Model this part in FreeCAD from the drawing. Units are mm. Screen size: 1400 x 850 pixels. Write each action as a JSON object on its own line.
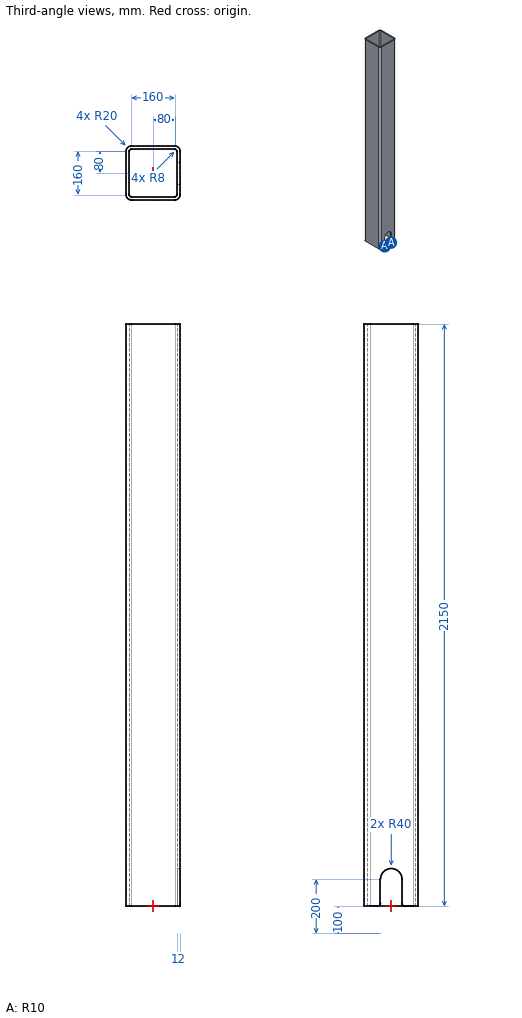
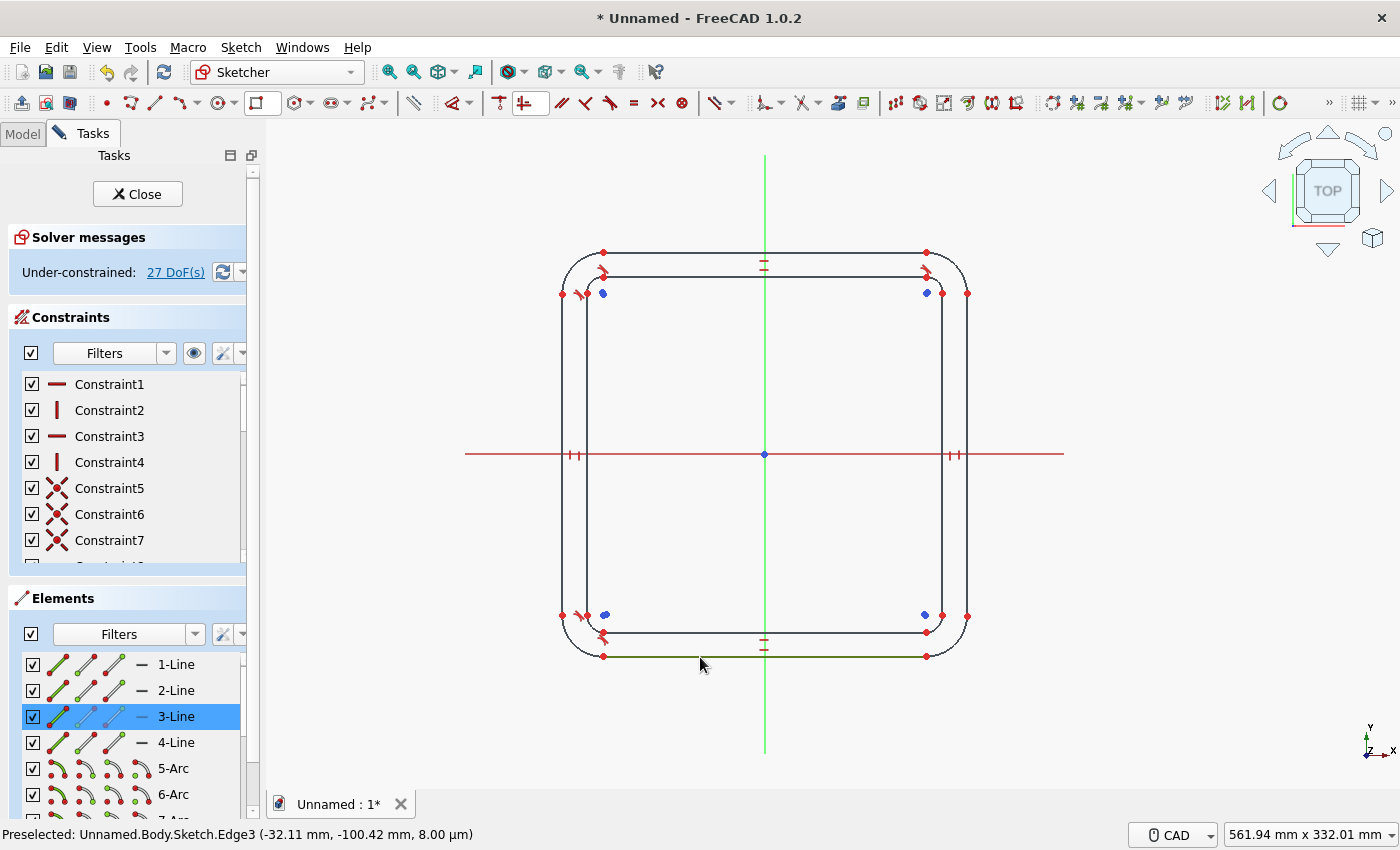
{"action": "left_click", "coordinate": [944, 652]}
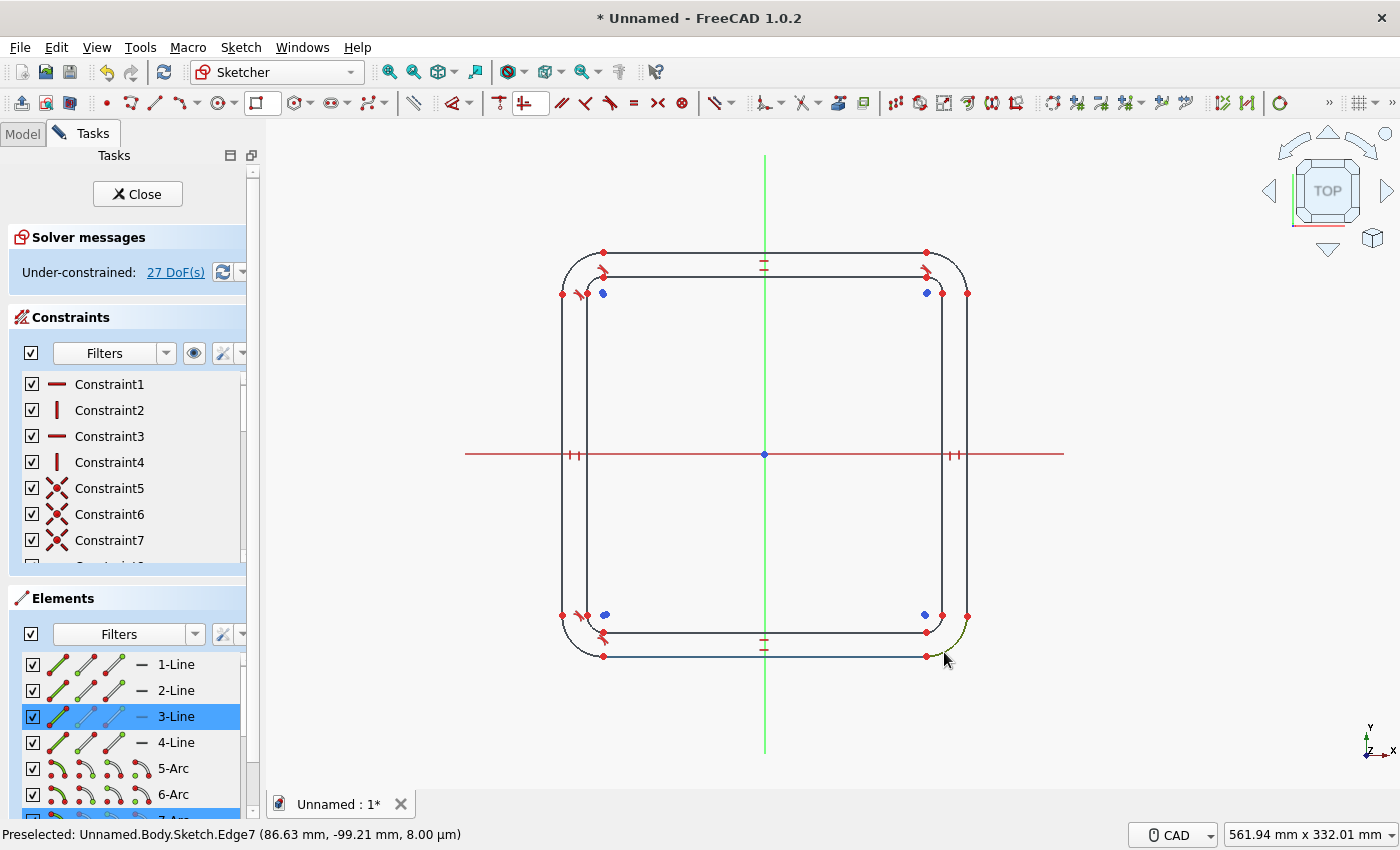
{"action": "left_click", "coordinate": [610, 104]}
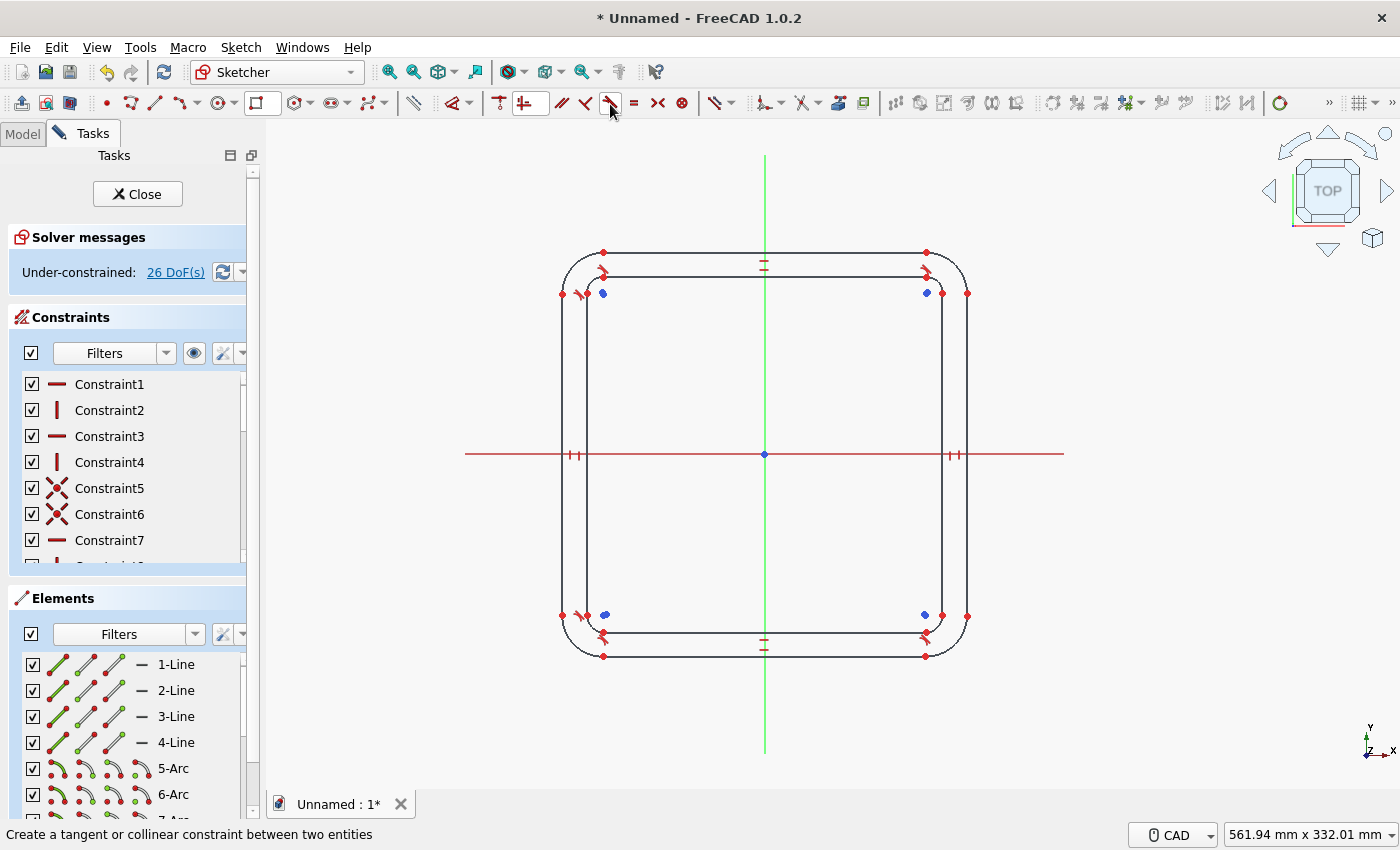
{"action": "left_click", "coordinate": [967, 520]}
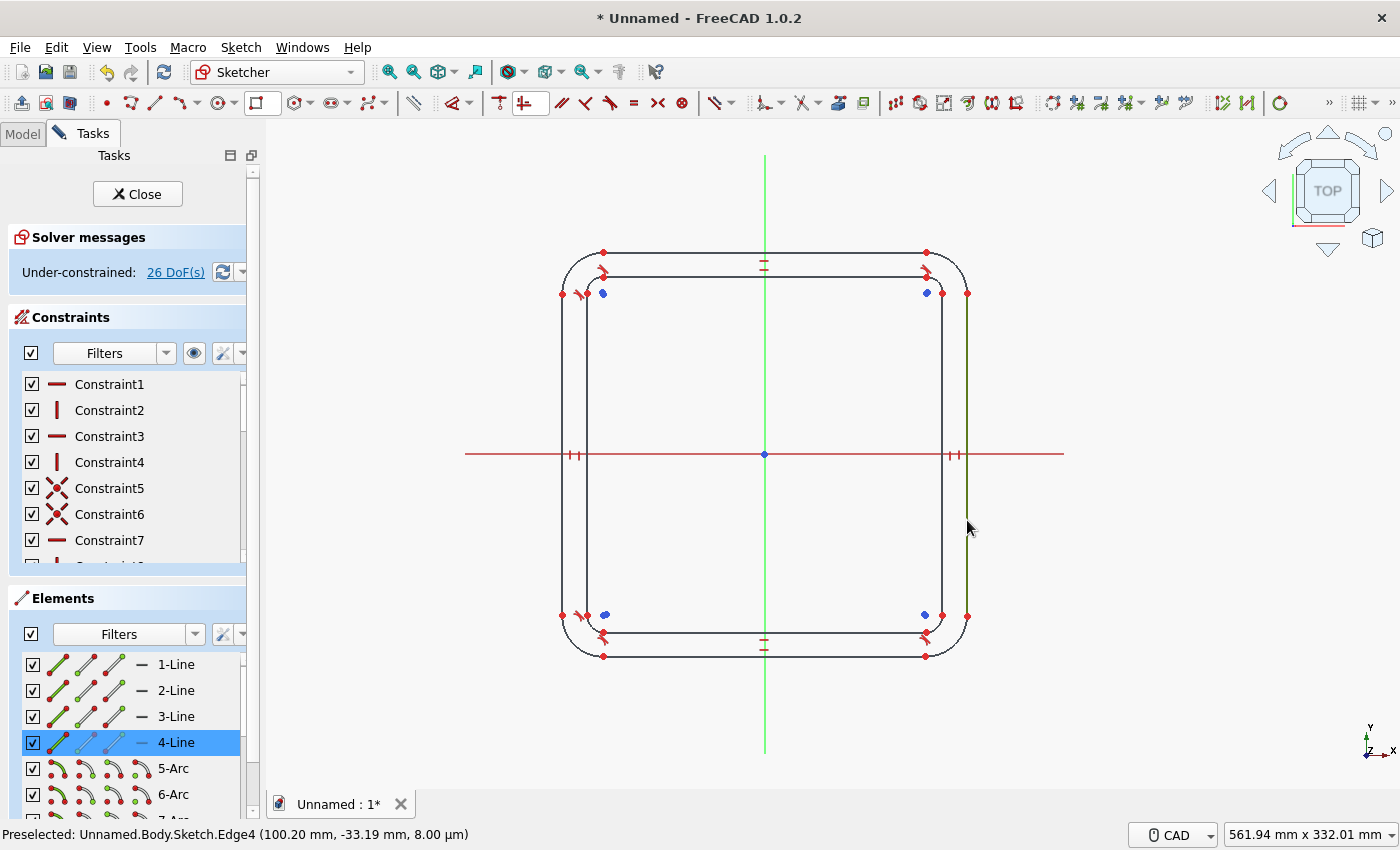
{"action": "left_click", "coordinate": [944, 652]}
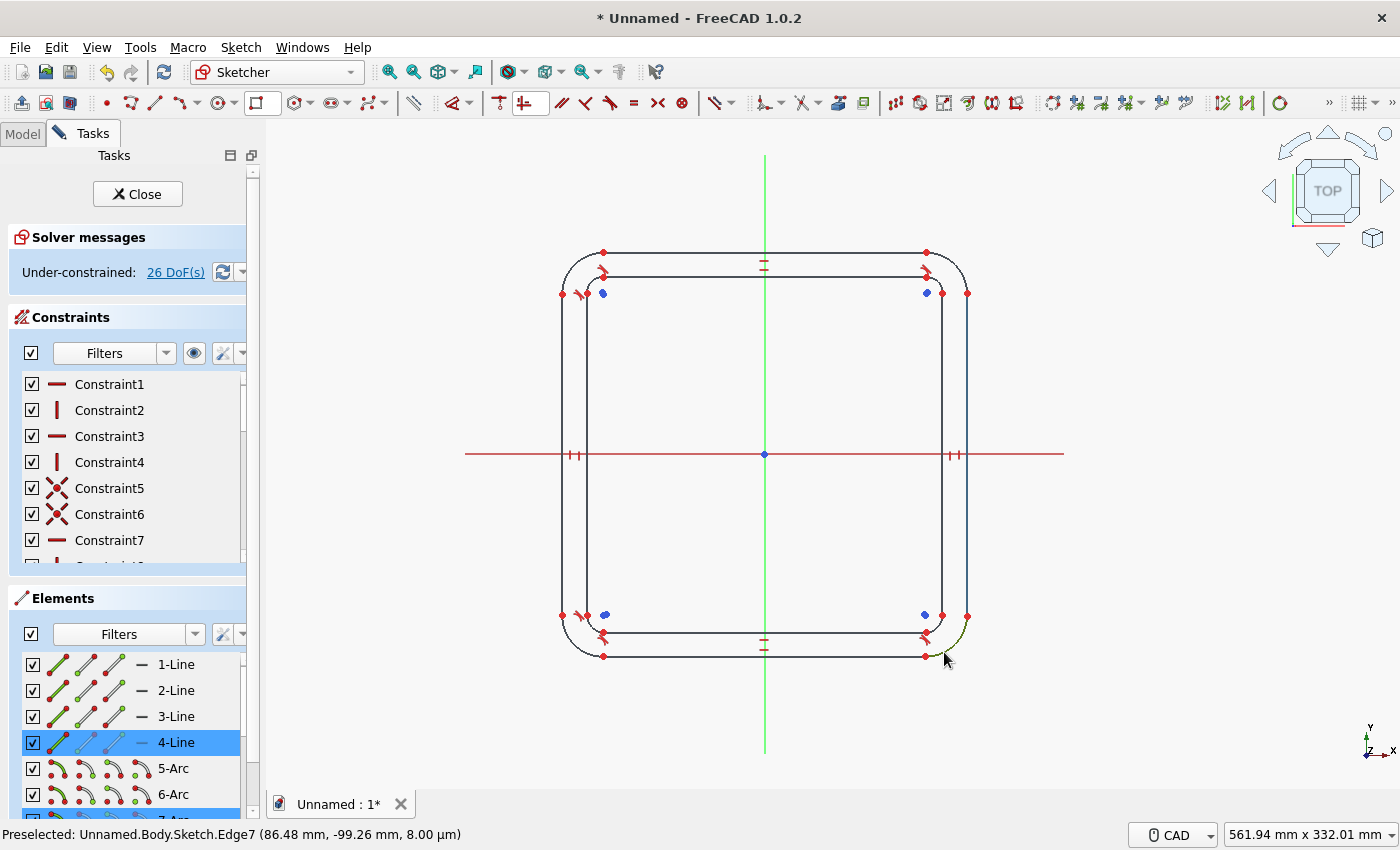
{"action": "left_click", "coordinate": [610, 104]}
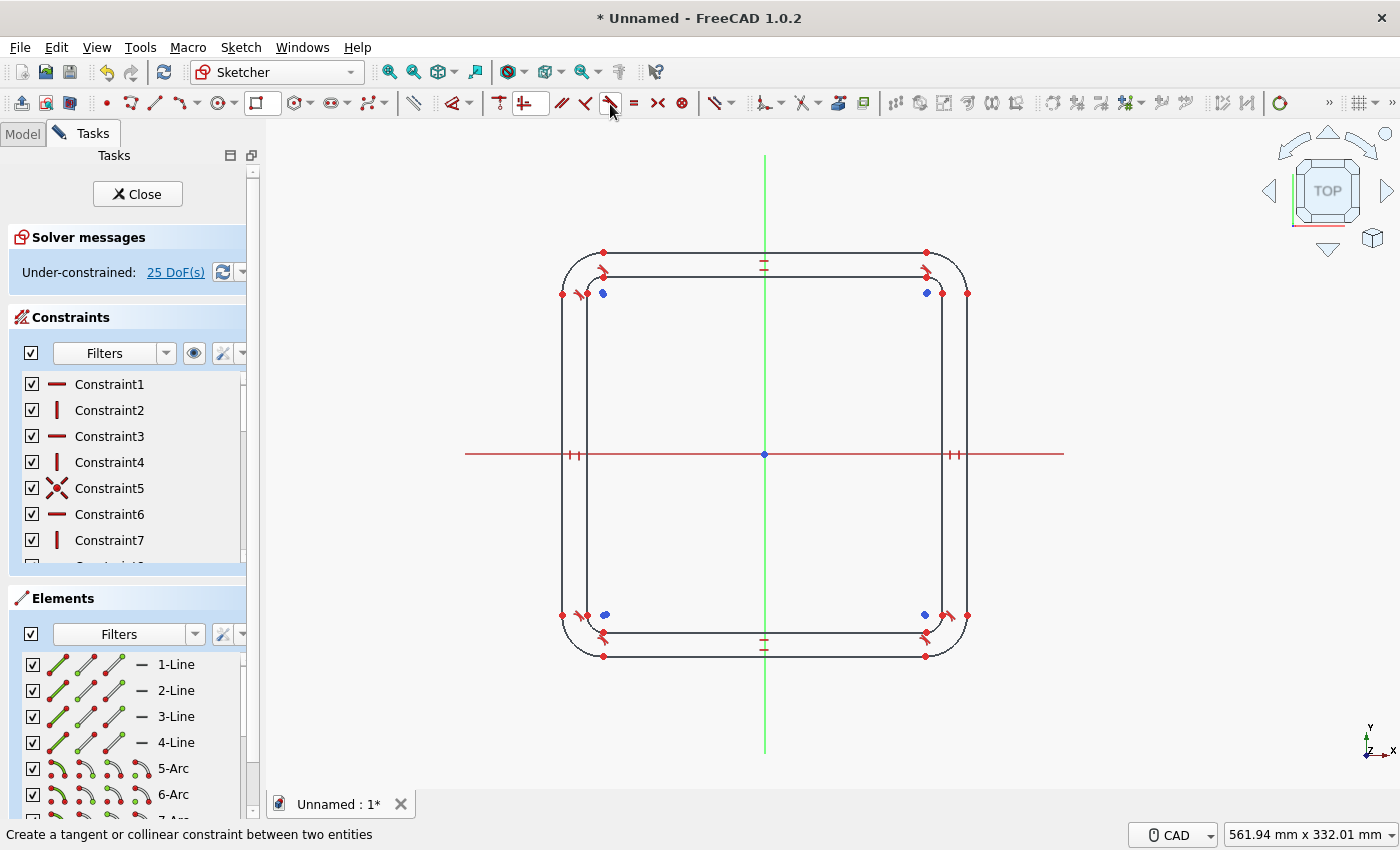
{"action": "left_click", "coordinate": [967, 519]}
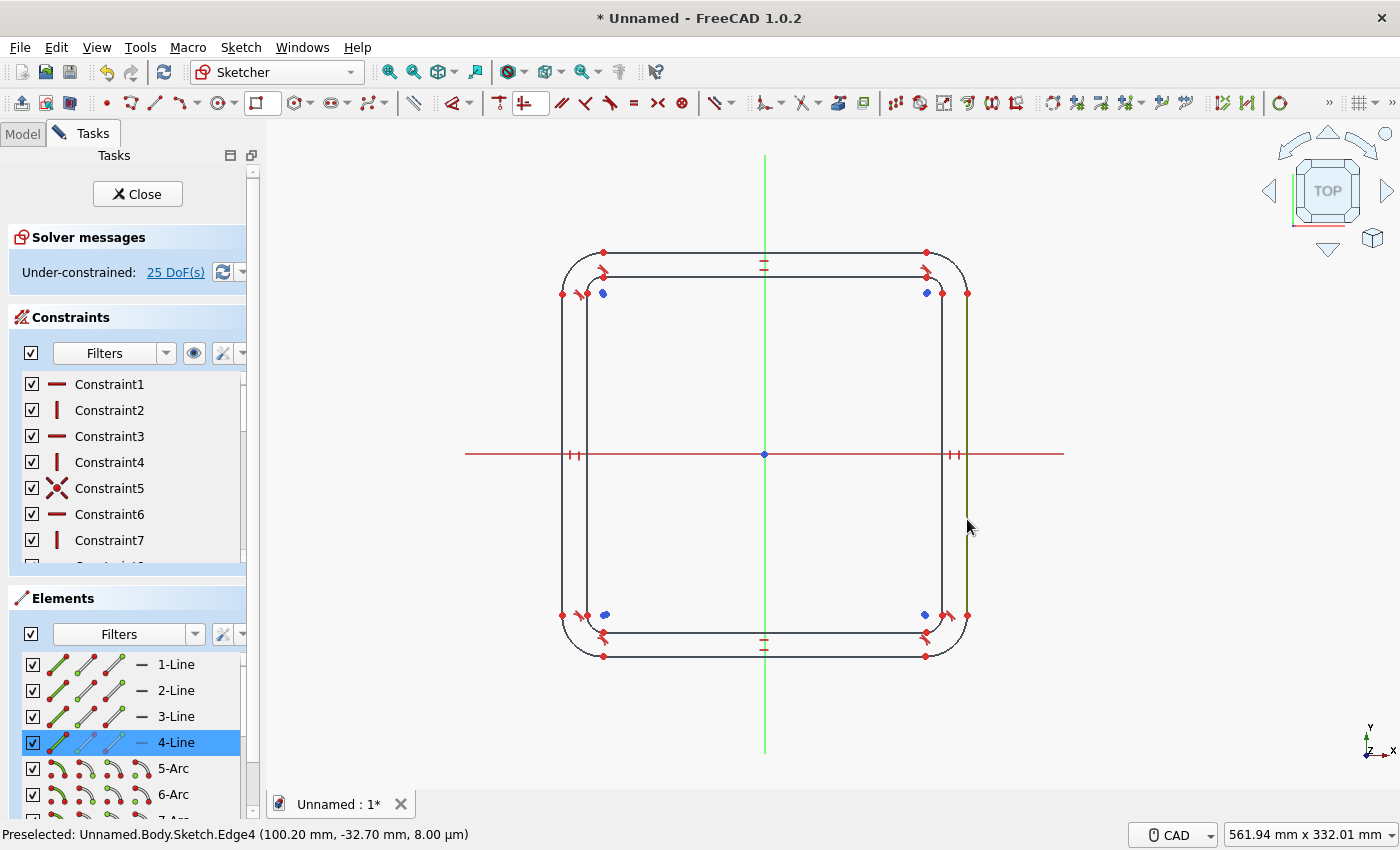
{"action": "left_click", "coordinate": [963, 275]}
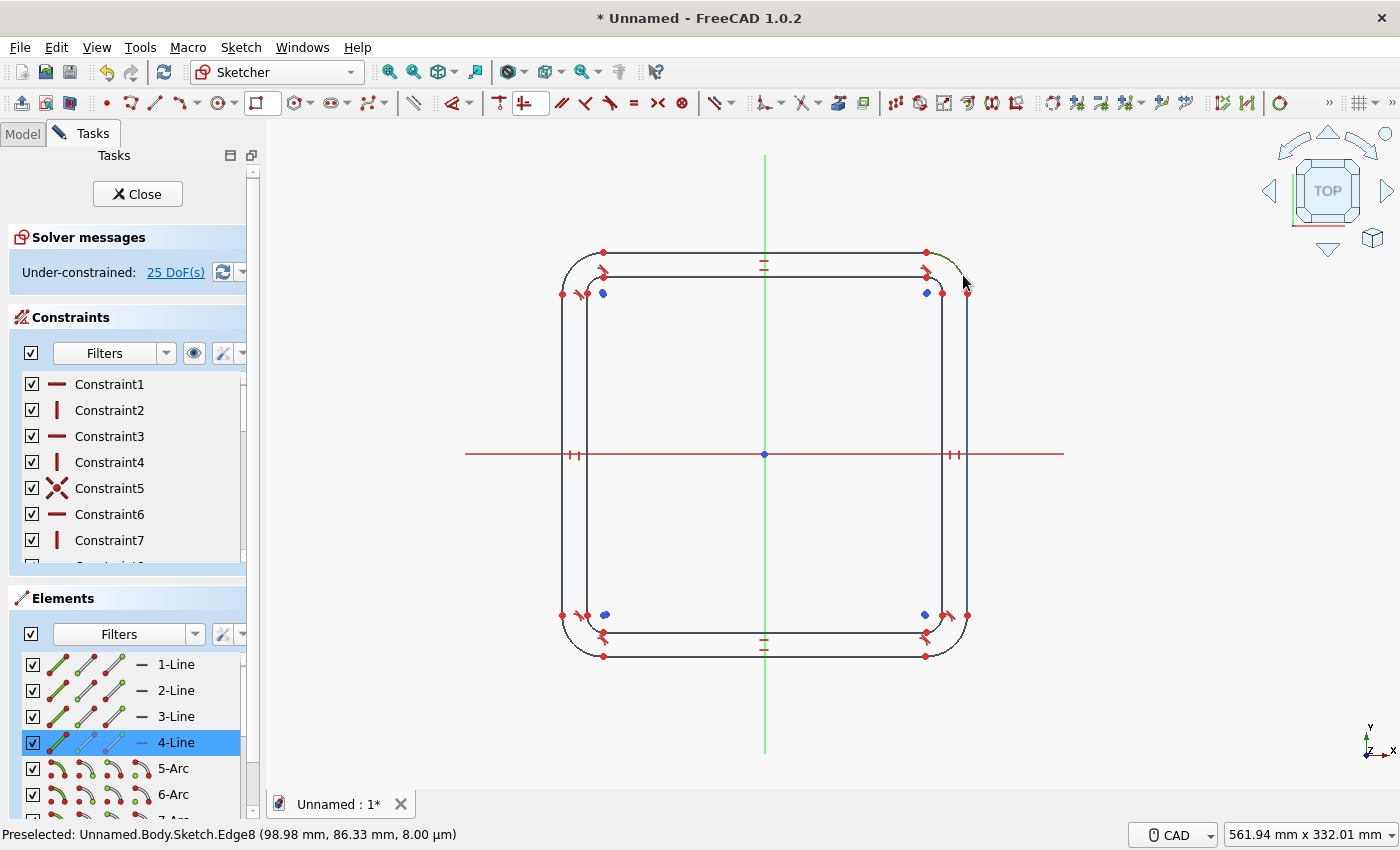
{"action": "left_click", "coordinate": [610, 104]}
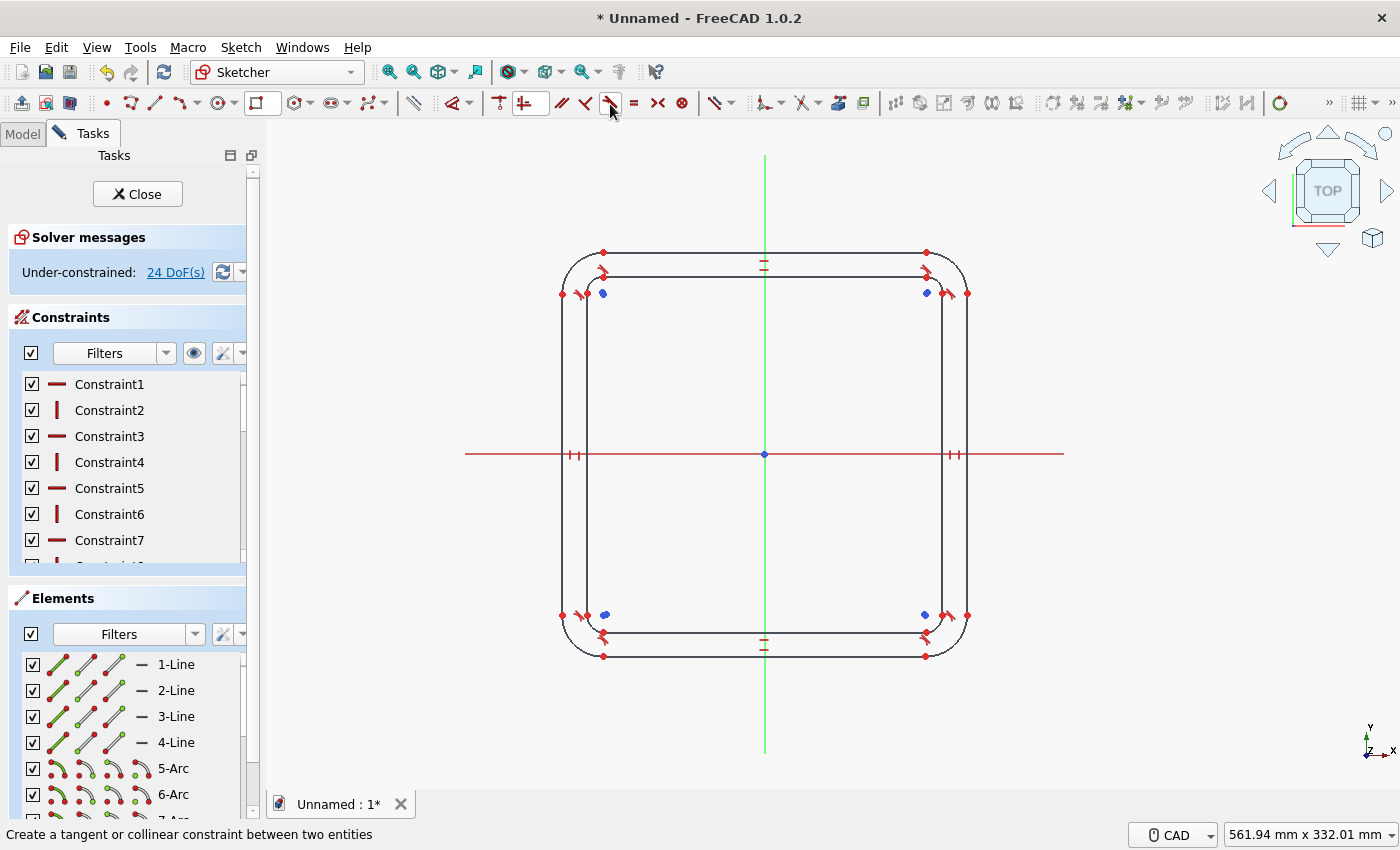
{"action": "left_click", "coordinate": [700, 277]}